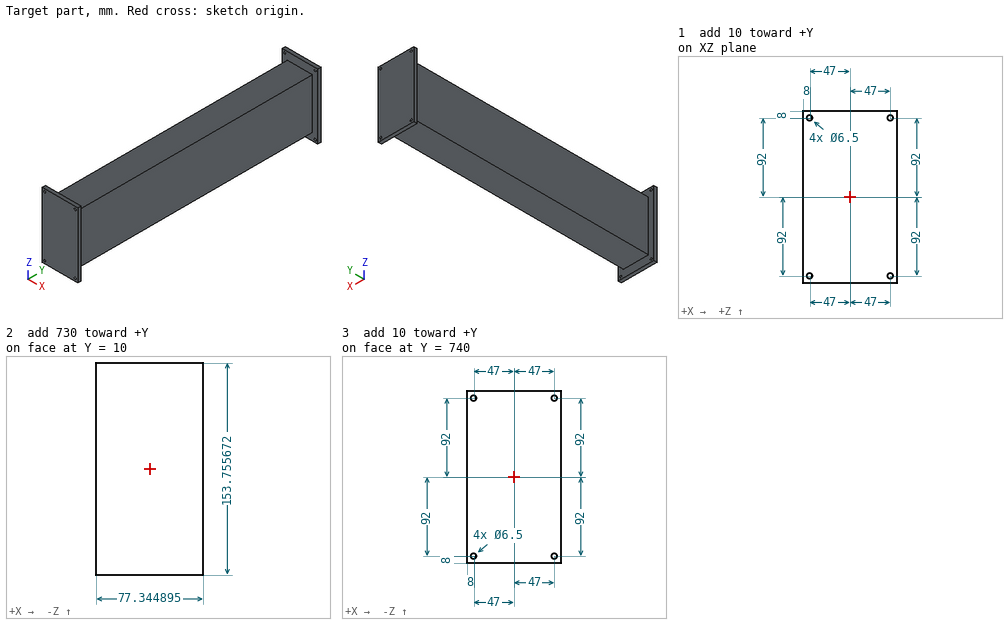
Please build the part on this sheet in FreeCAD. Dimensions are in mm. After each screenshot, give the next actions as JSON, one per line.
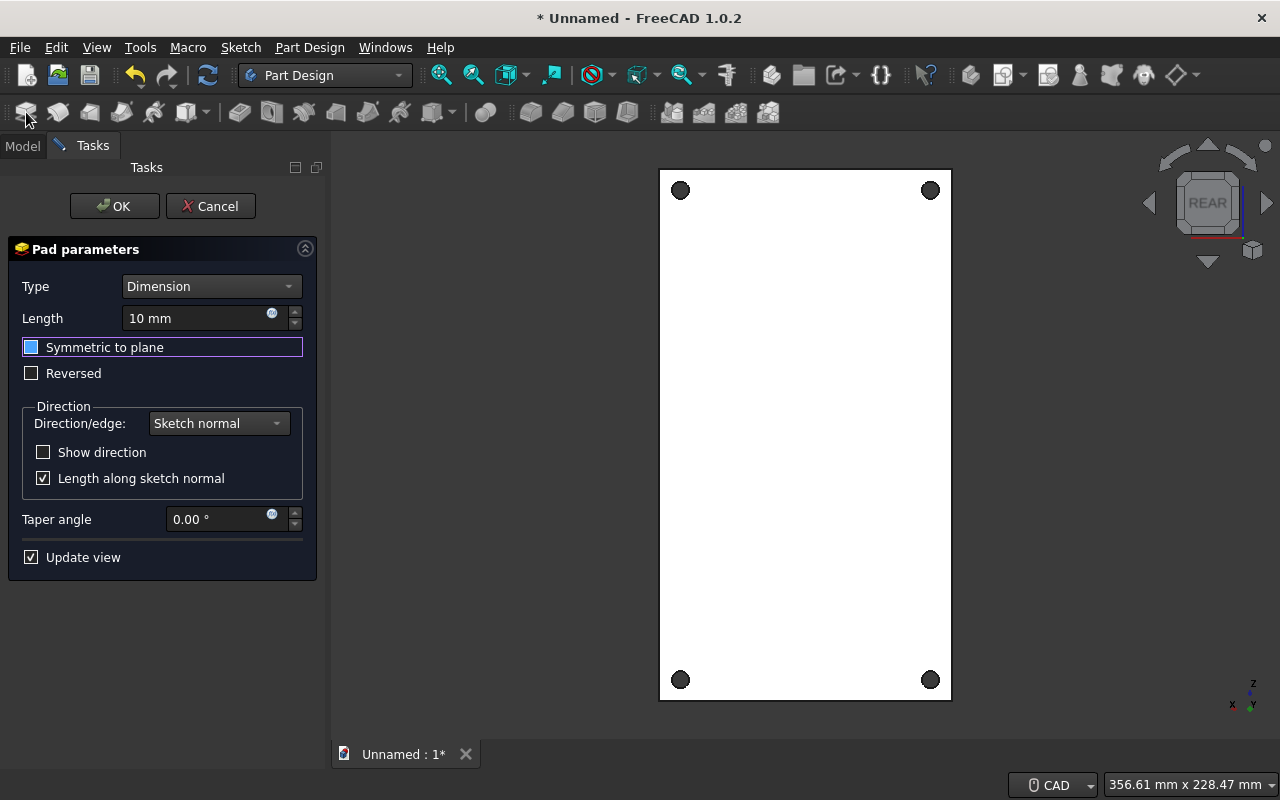
{"action": "left_click", "coordinate": [115, 206]}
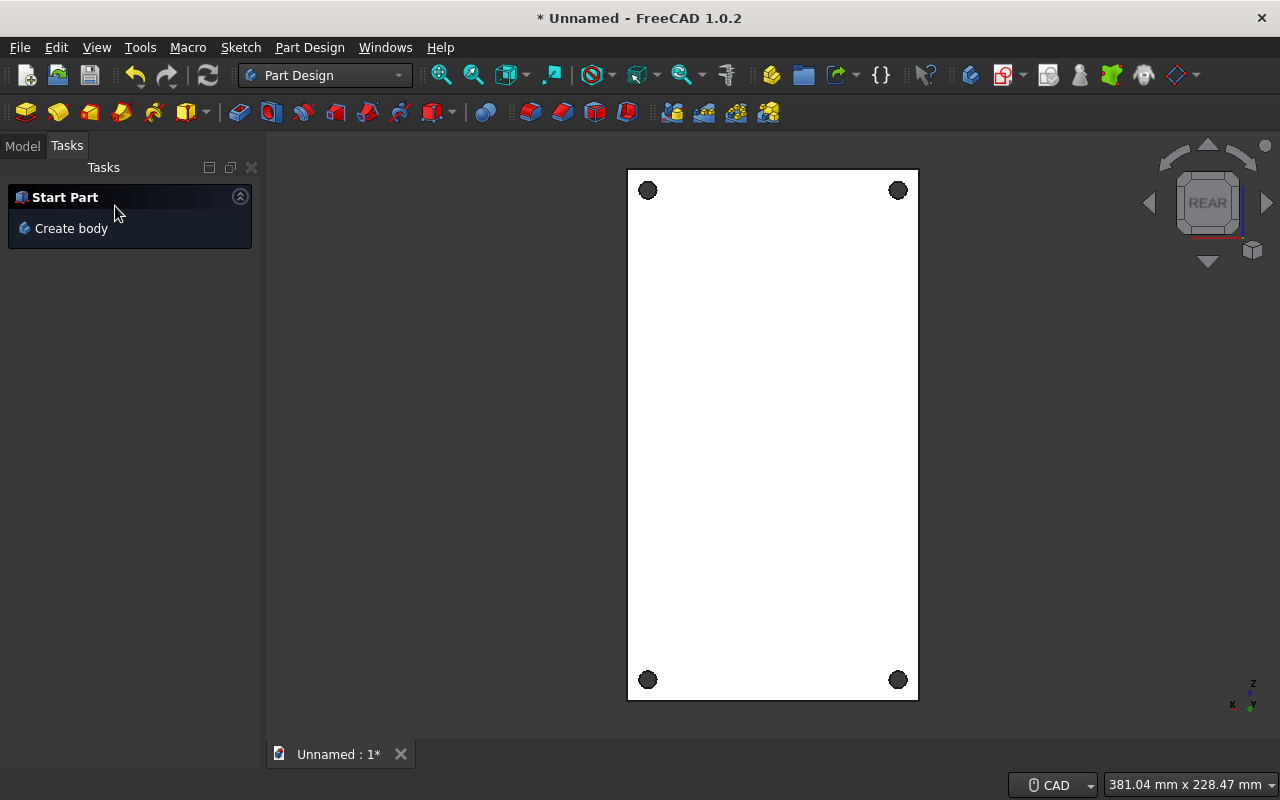
{"action": "key", "text": "0"}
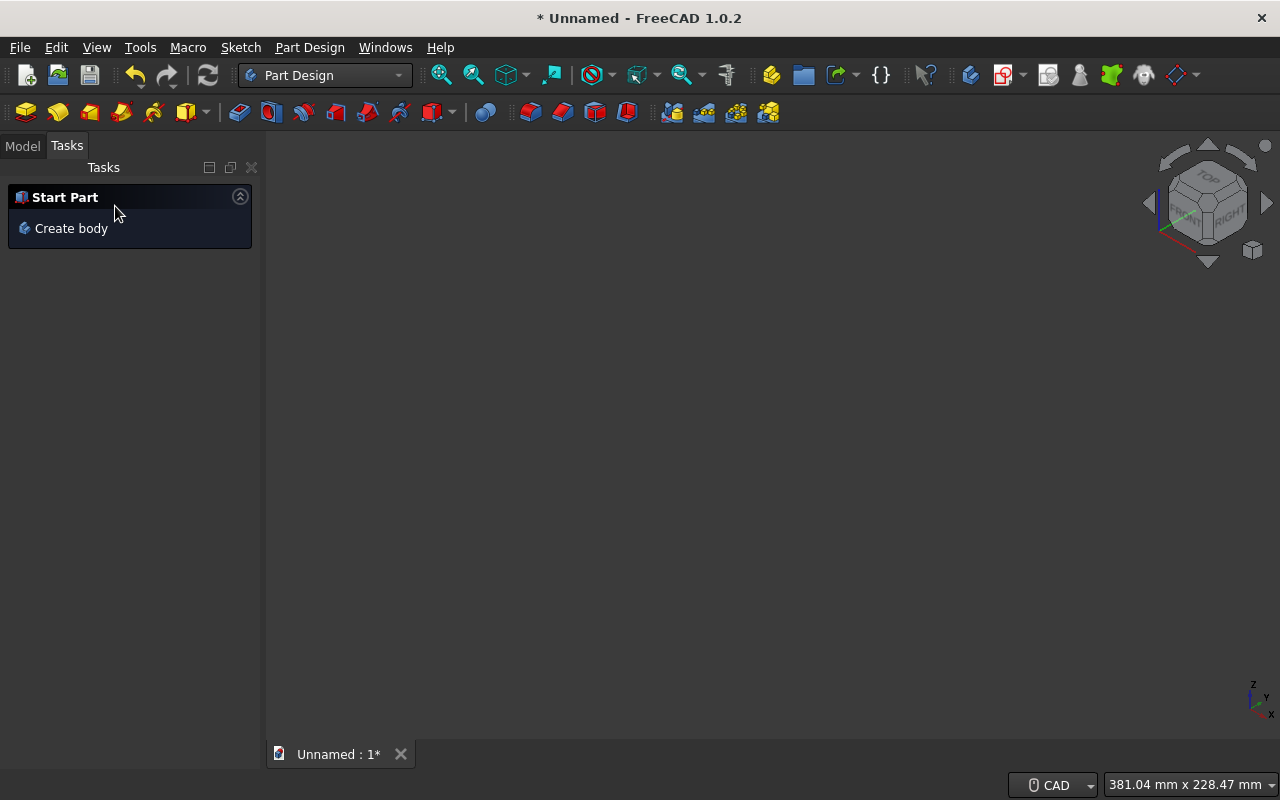
{"action": "left_click", "coordinate": [442, 76]}